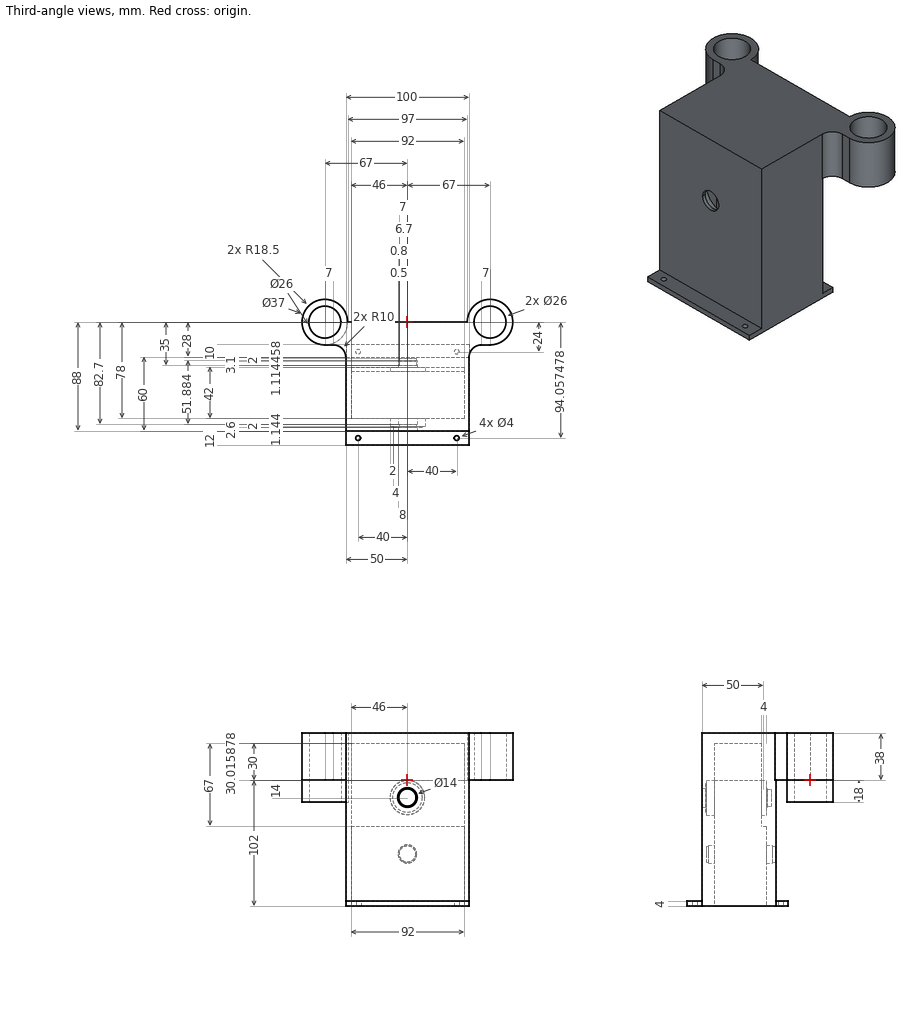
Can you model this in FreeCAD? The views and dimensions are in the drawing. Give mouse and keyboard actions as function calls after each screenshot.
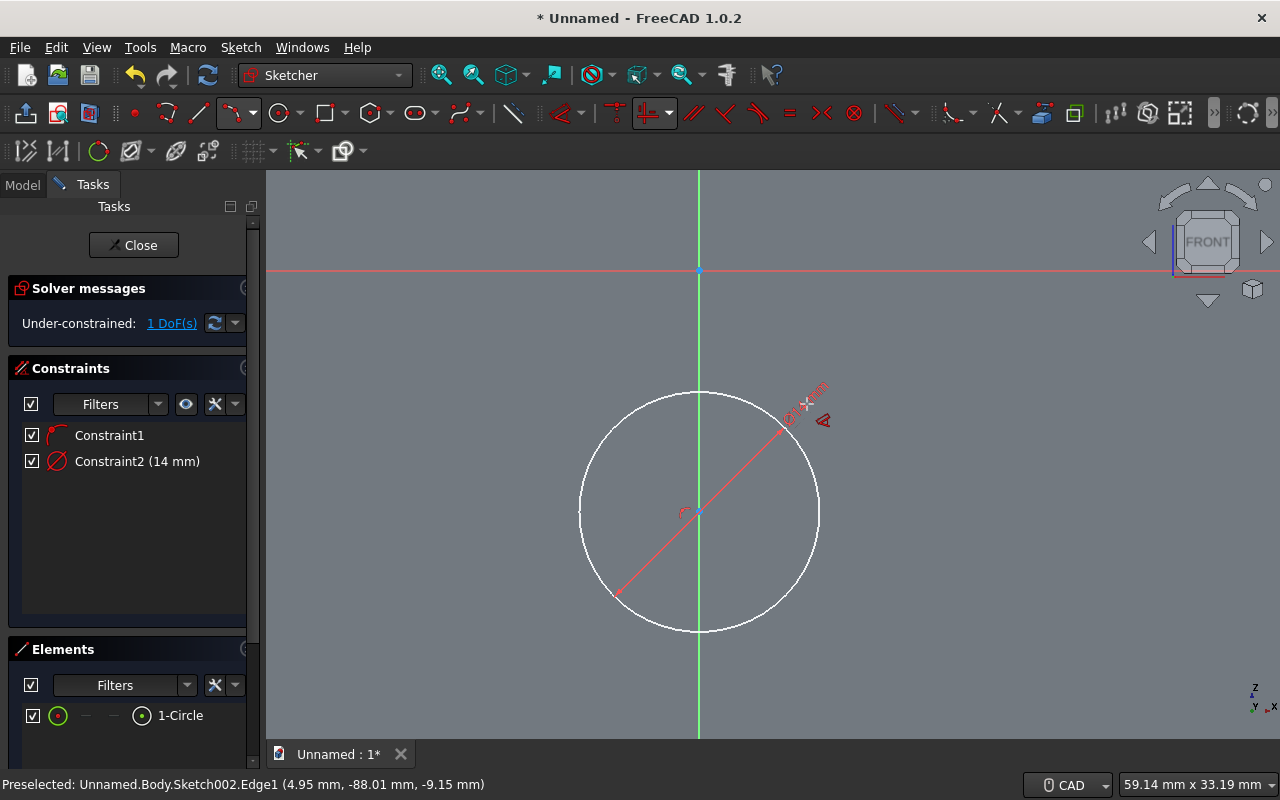
click(699, 512)
click(733, 336)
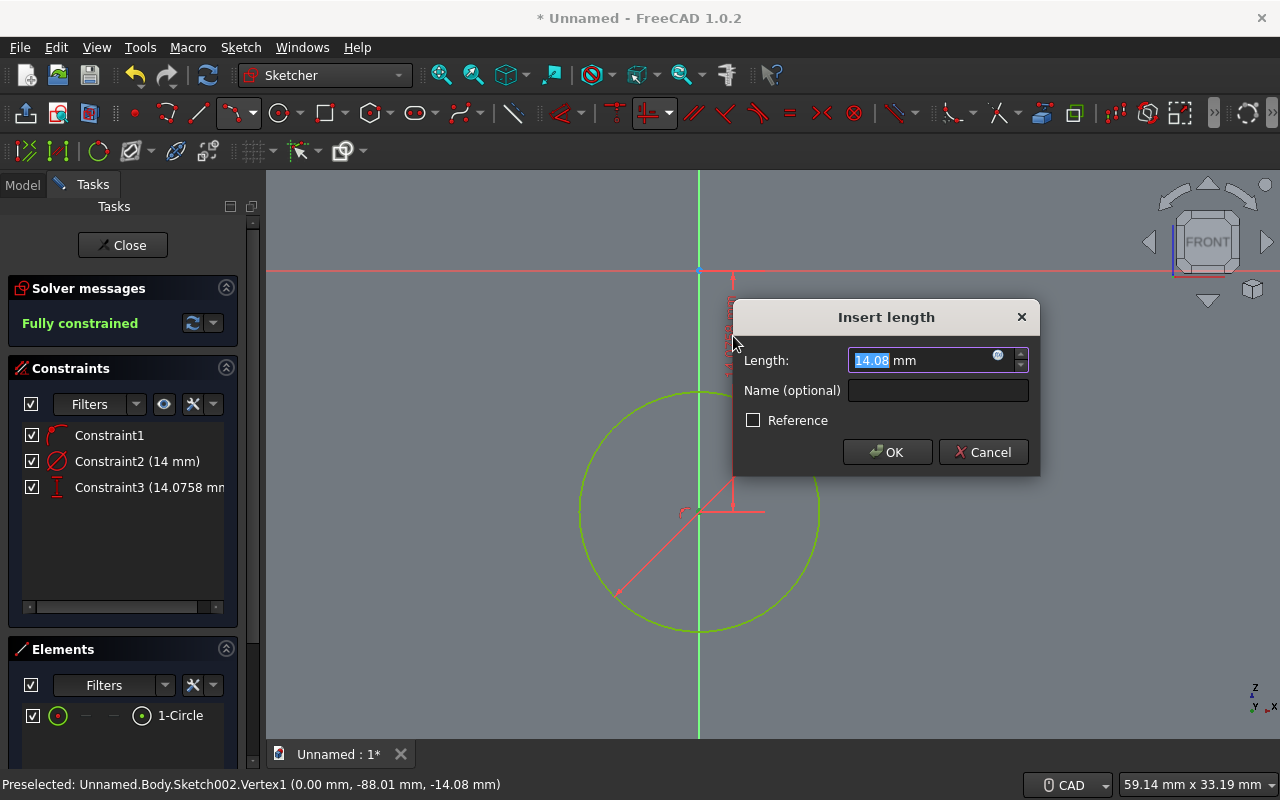
text(14)
key(Return)
key(Escape)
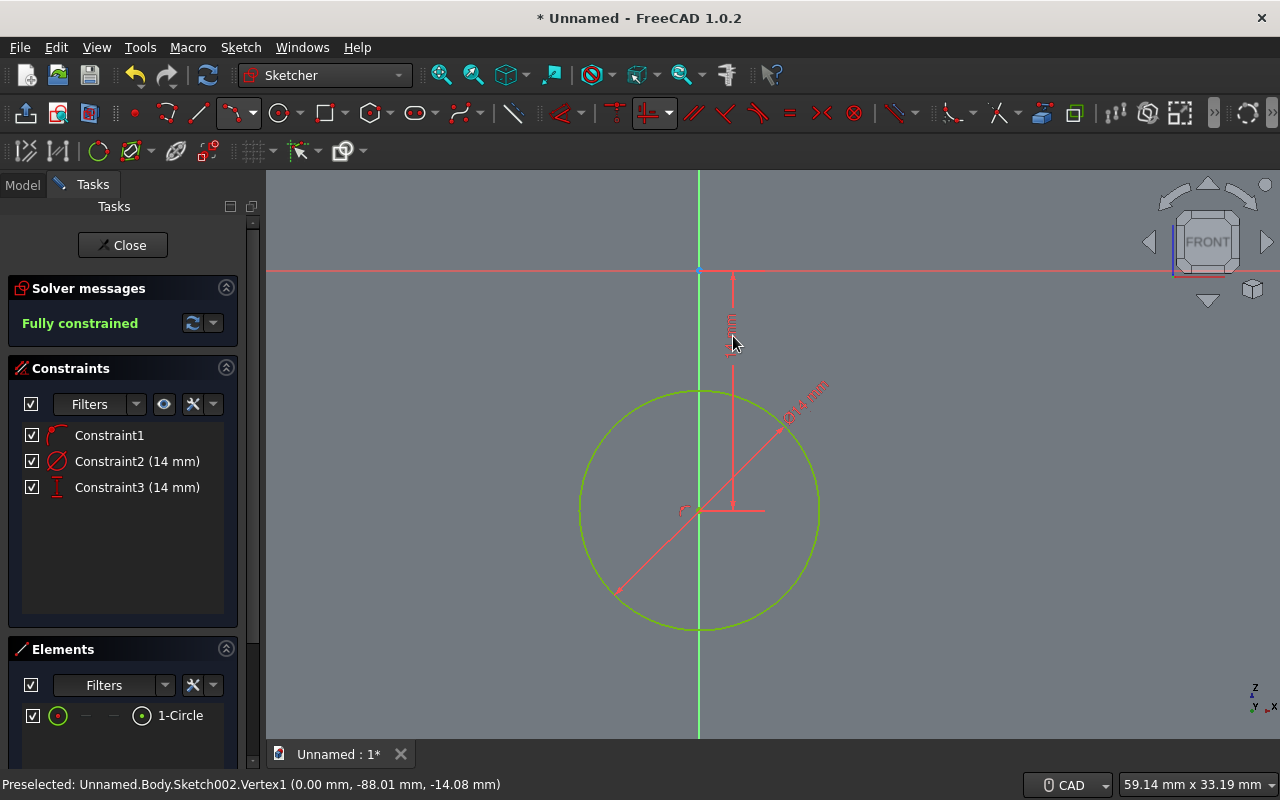
click(123, 245)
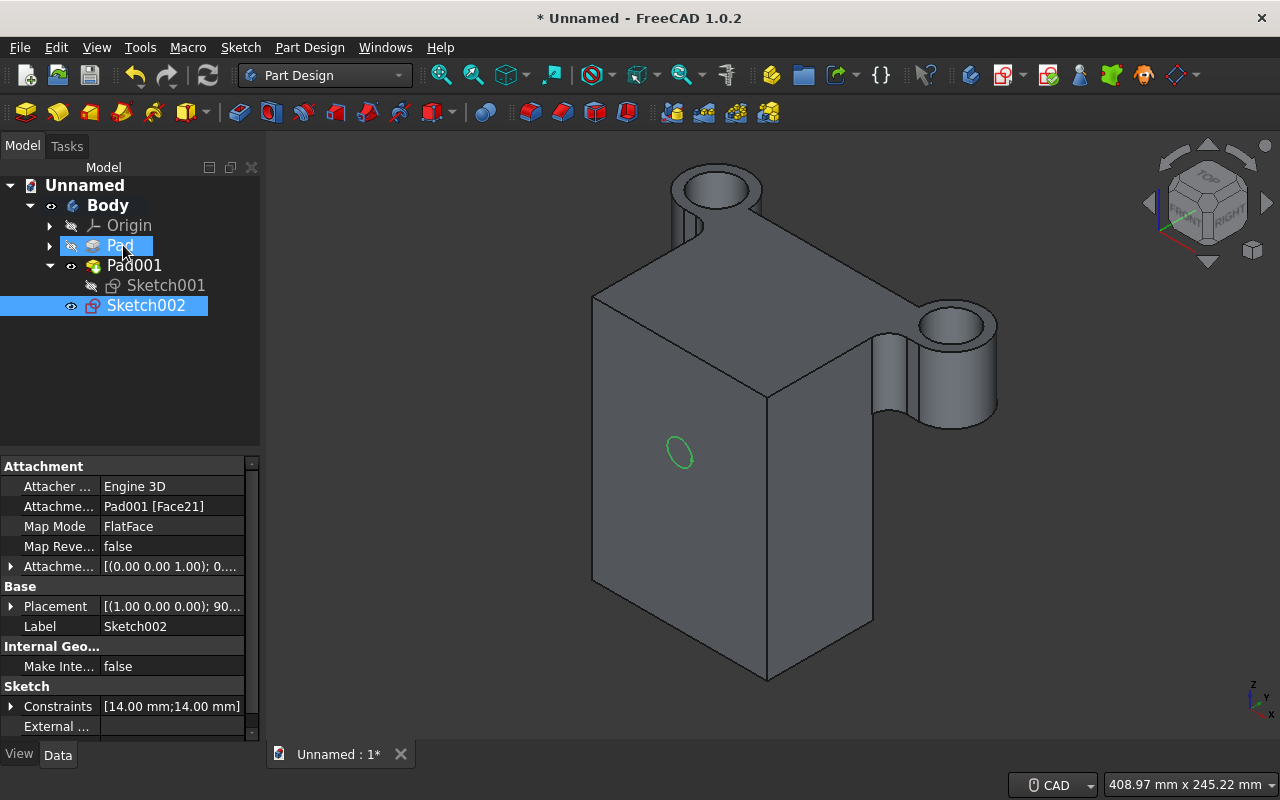
click(240, 112)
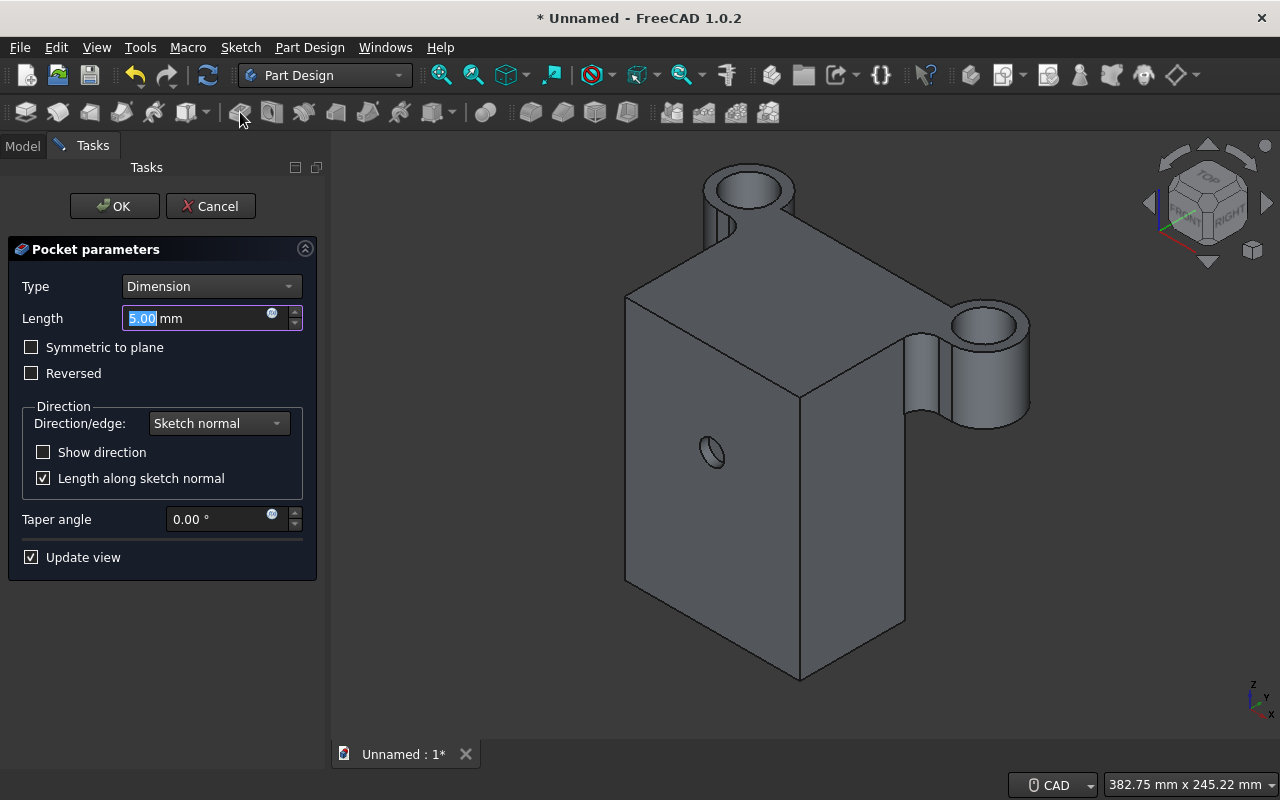
text(50)
key(Tab)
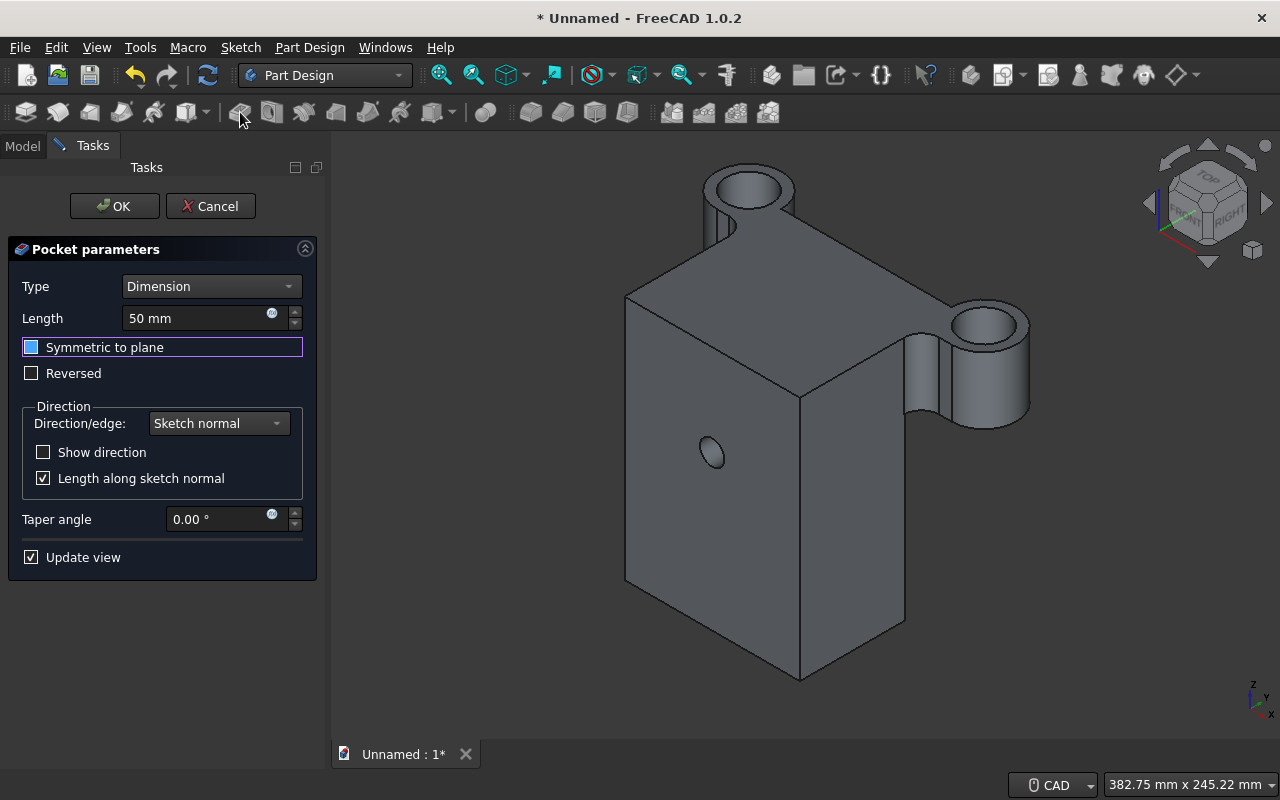
click(115, 206)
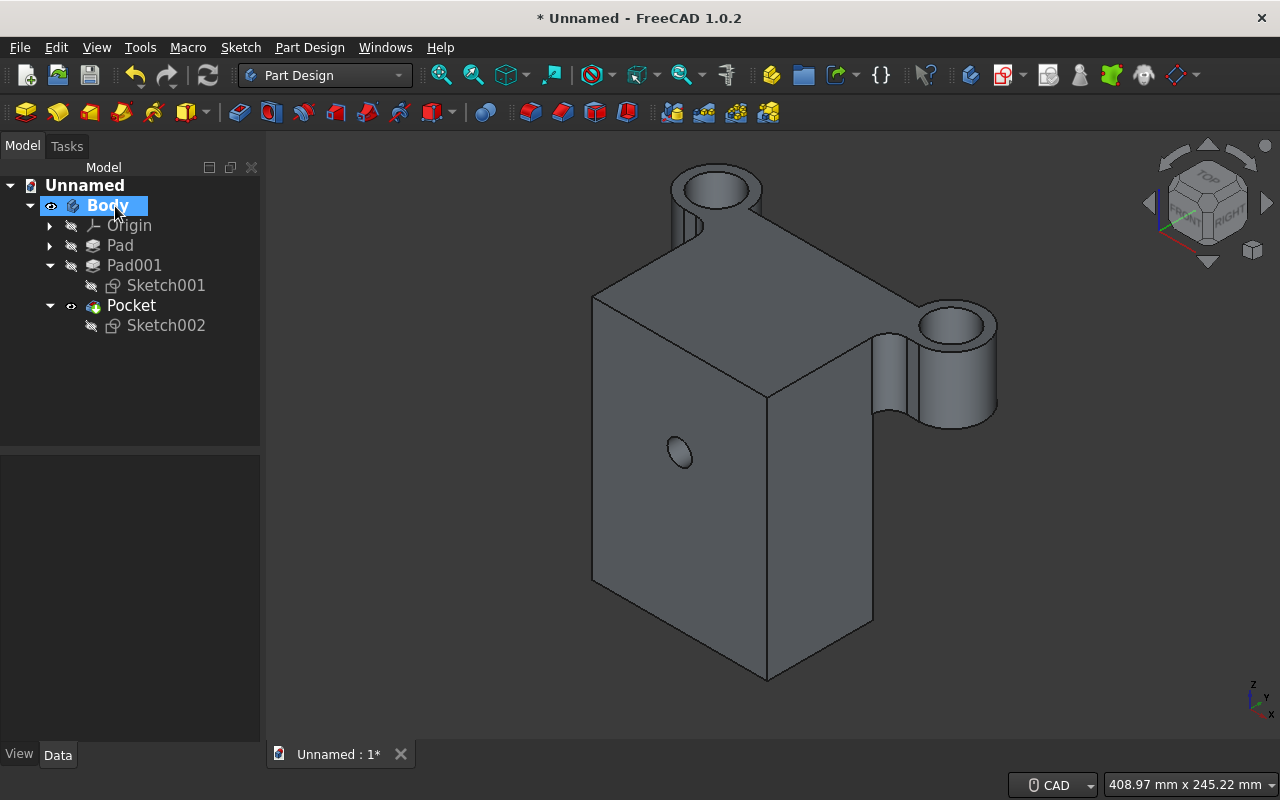
click(50, 226)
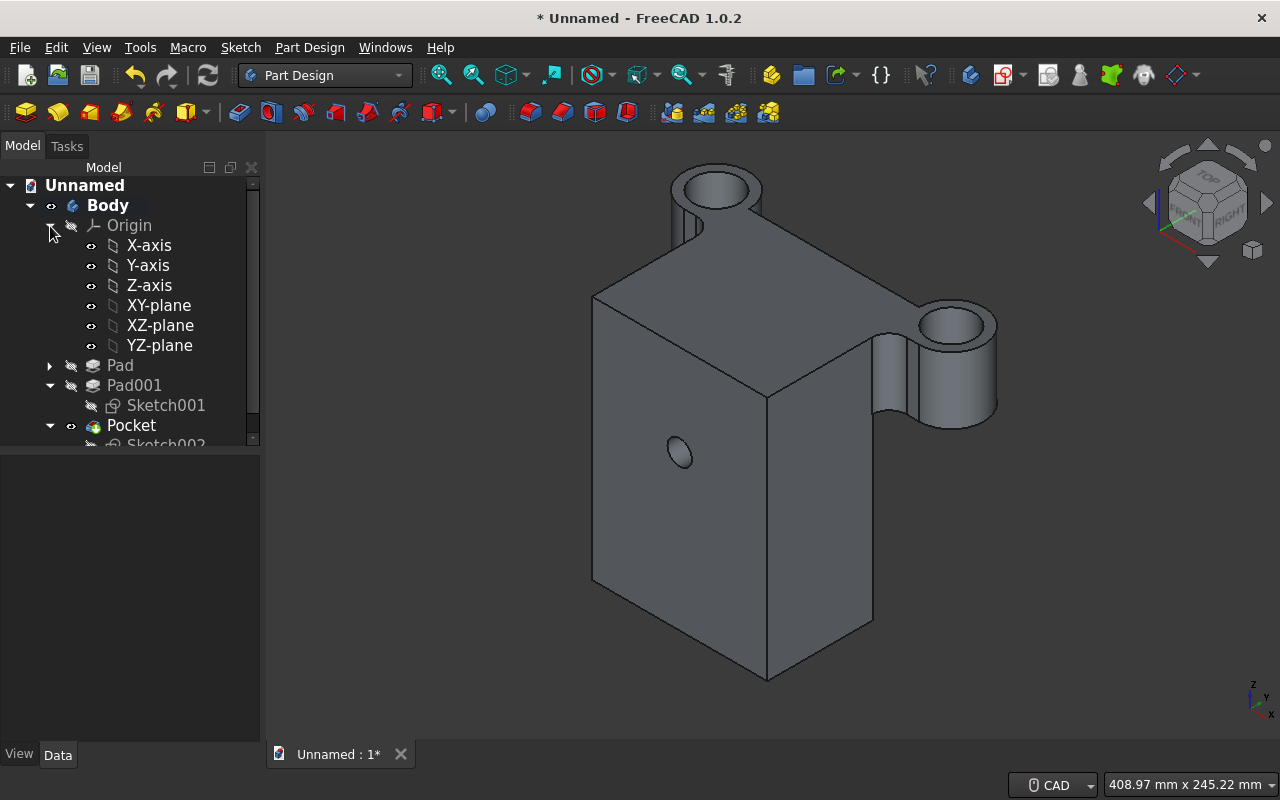
click(136, 306)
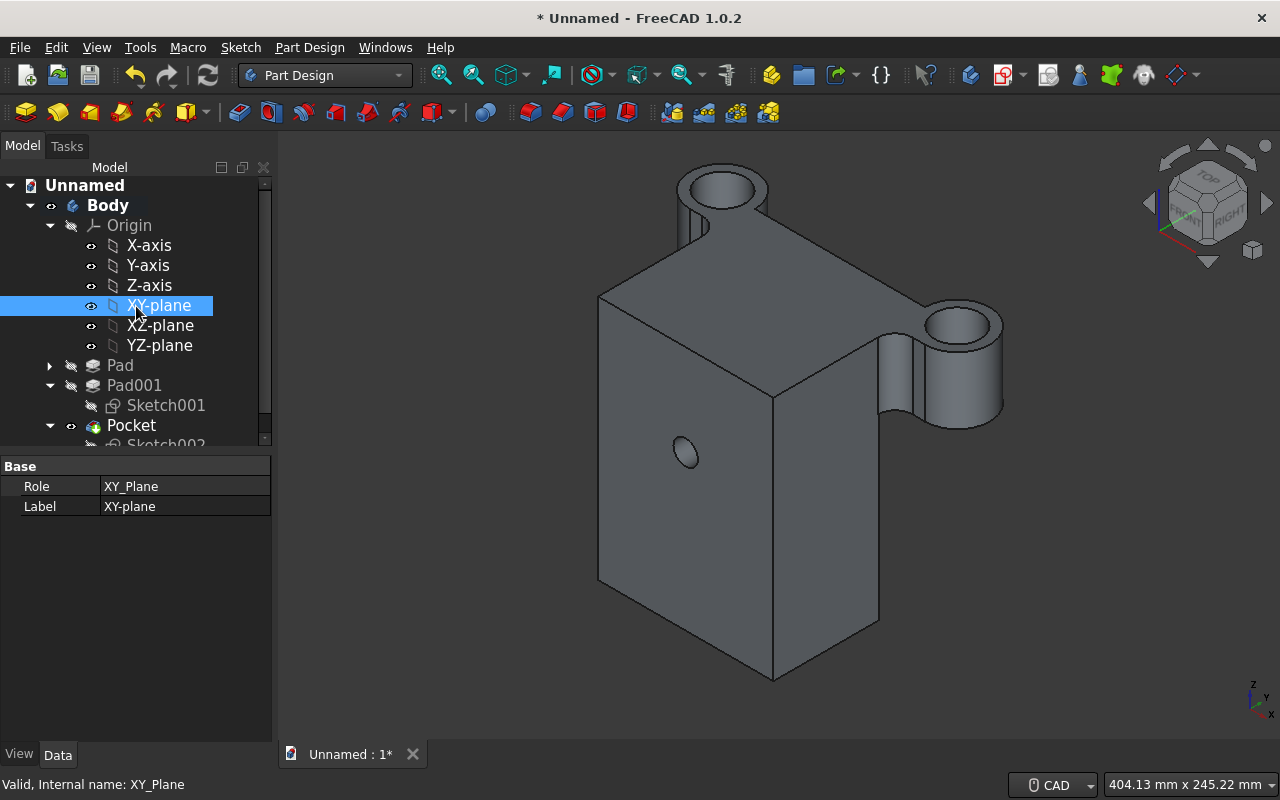
click(1176, 76)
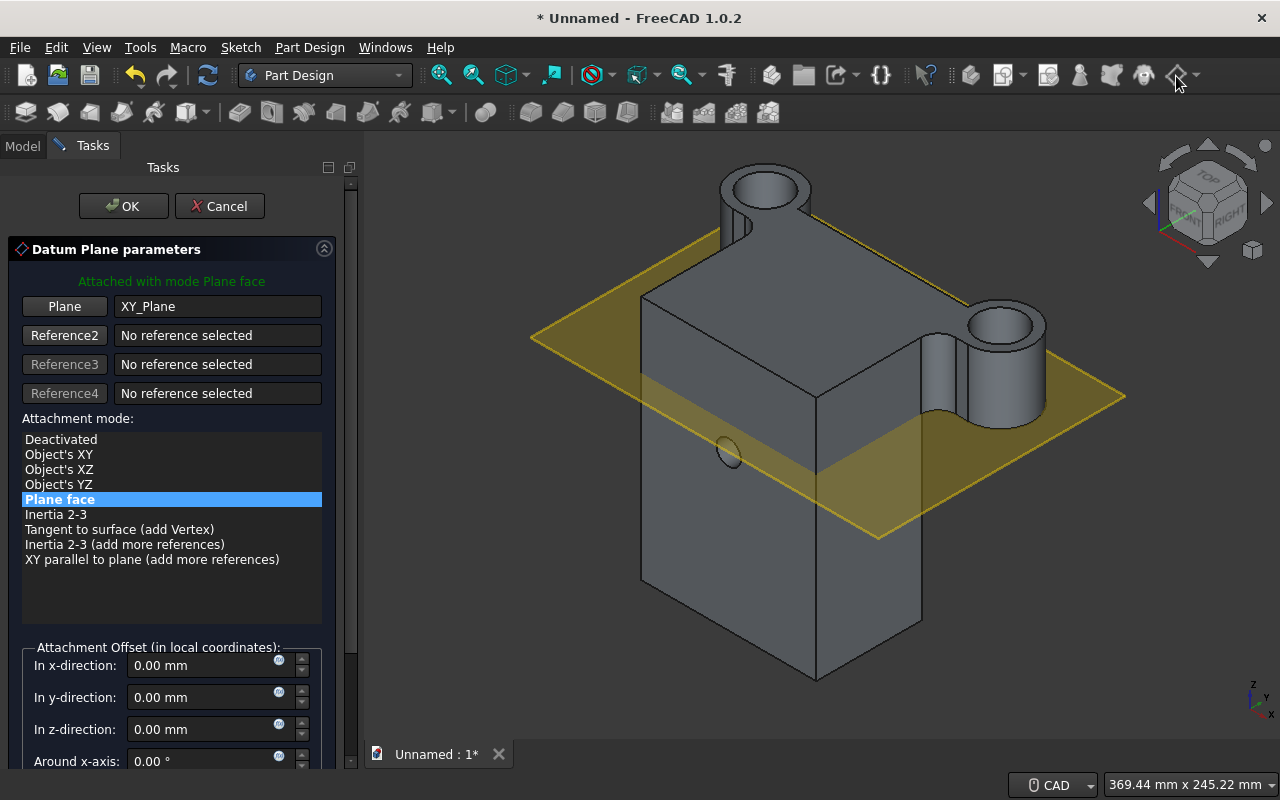
triple_click(210, 729)